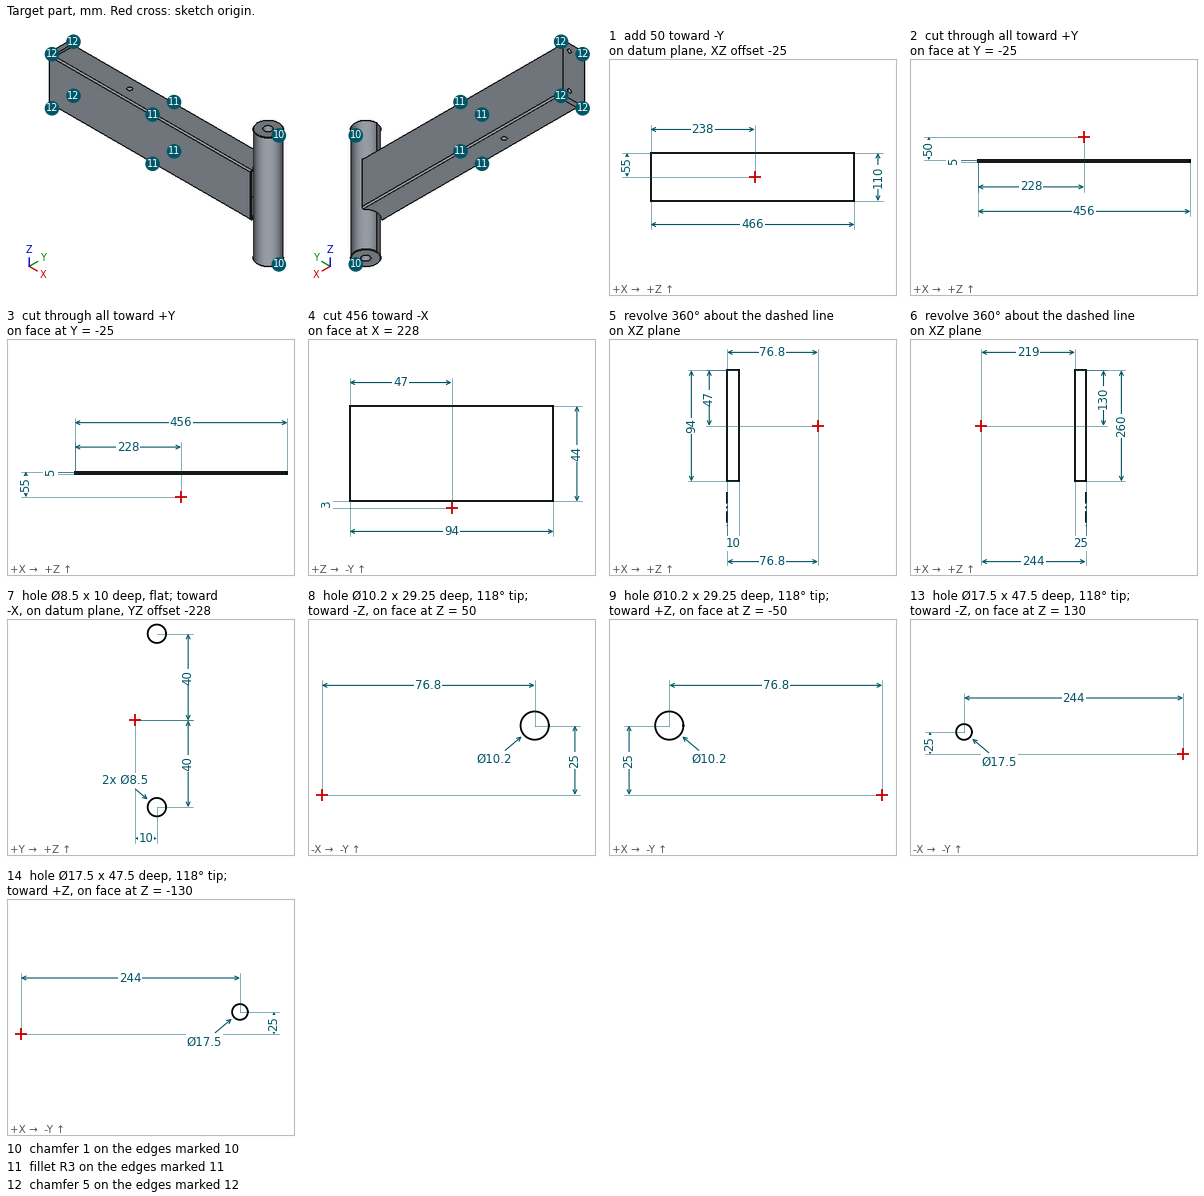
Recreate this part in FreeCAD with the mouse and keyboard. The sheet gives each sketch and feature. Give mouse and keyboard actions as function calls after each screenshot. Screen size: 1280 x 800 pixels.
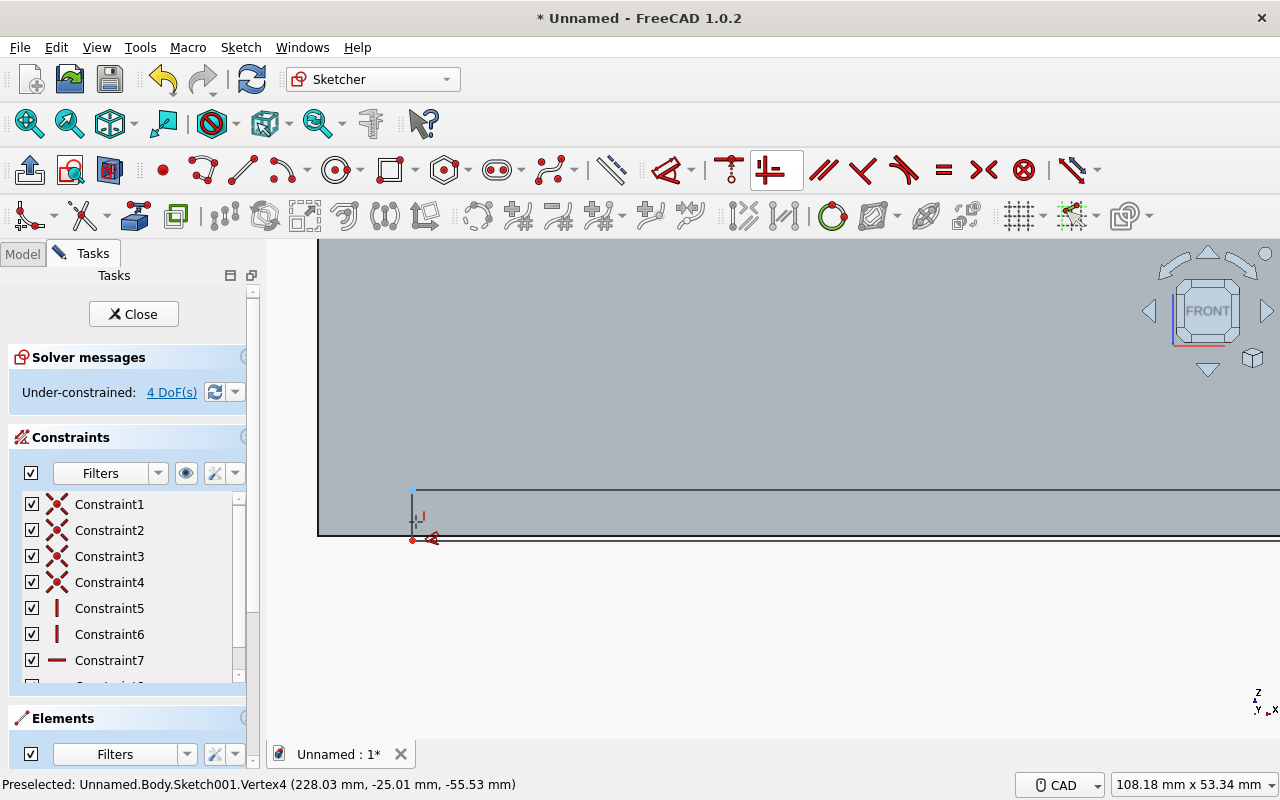
click(412, 515)
click(378, 515)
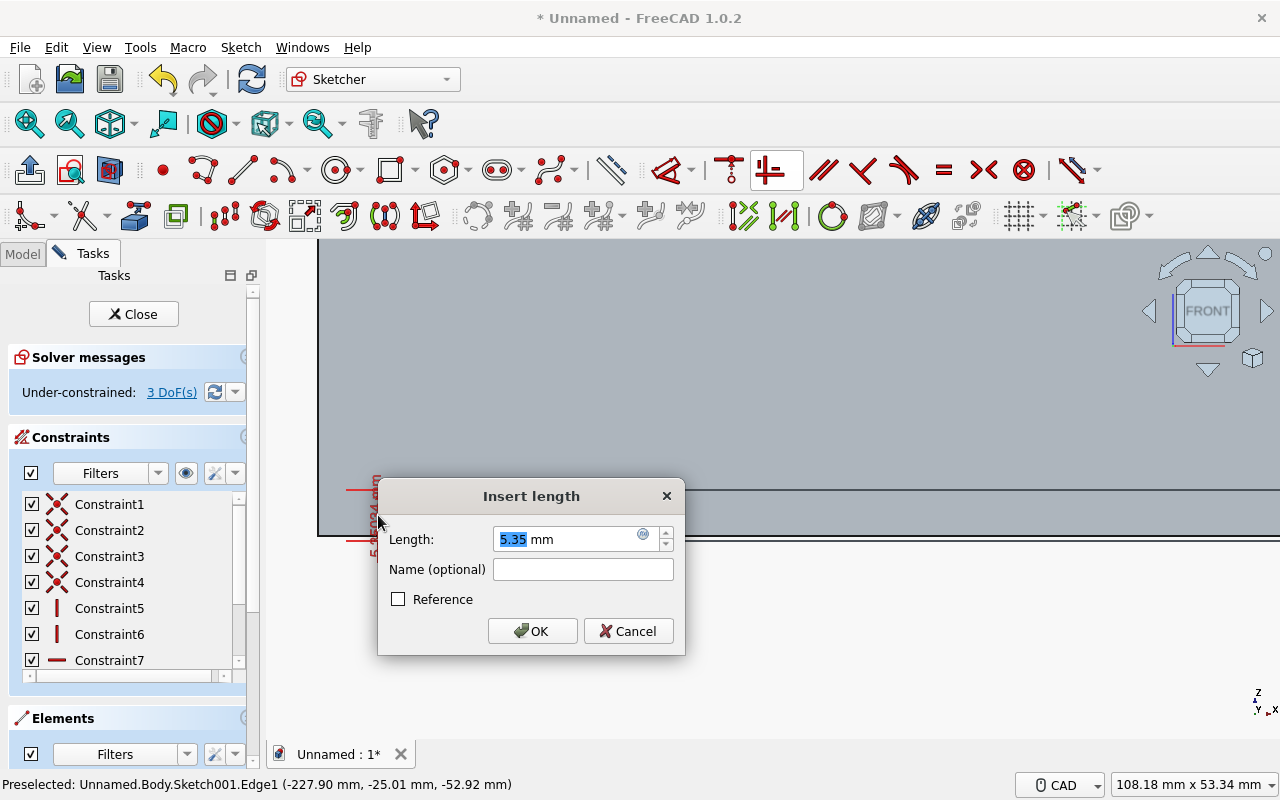
text(5)
key(Return)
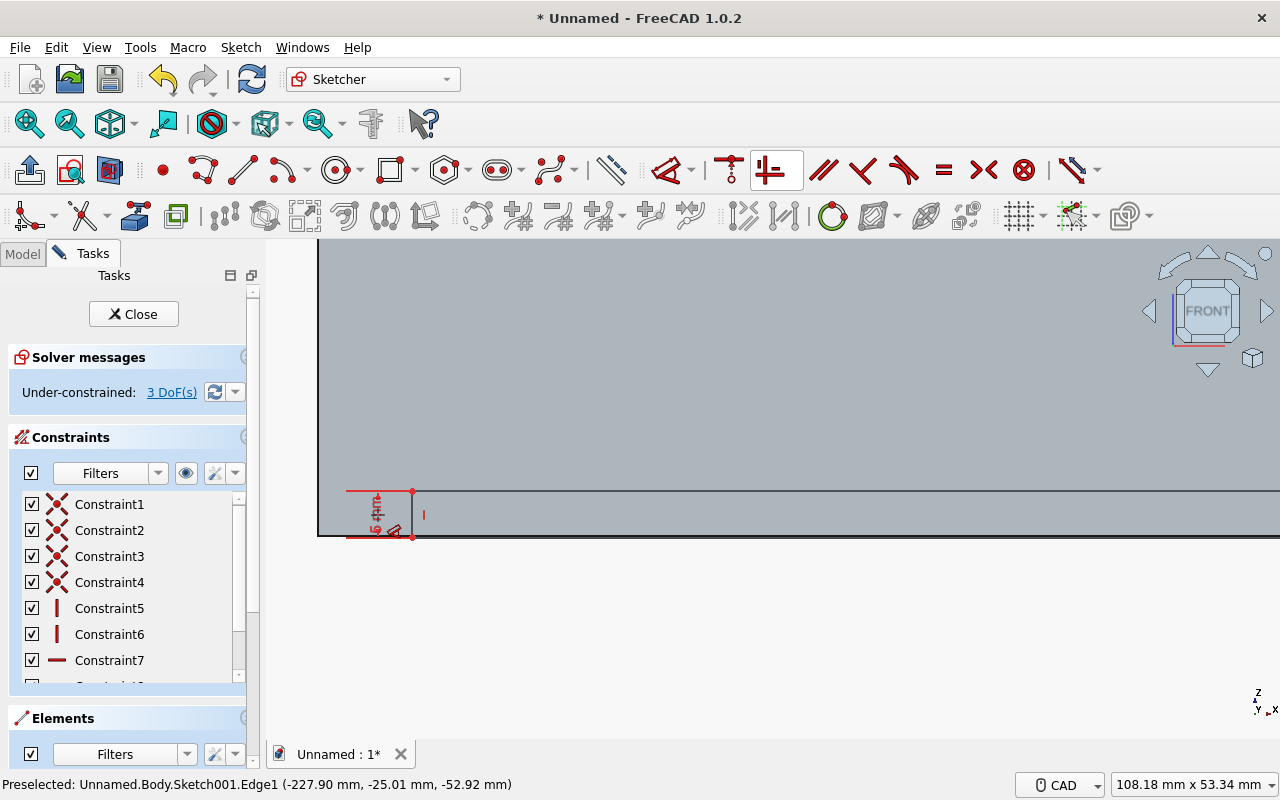
scroll(416, 522, down, 10)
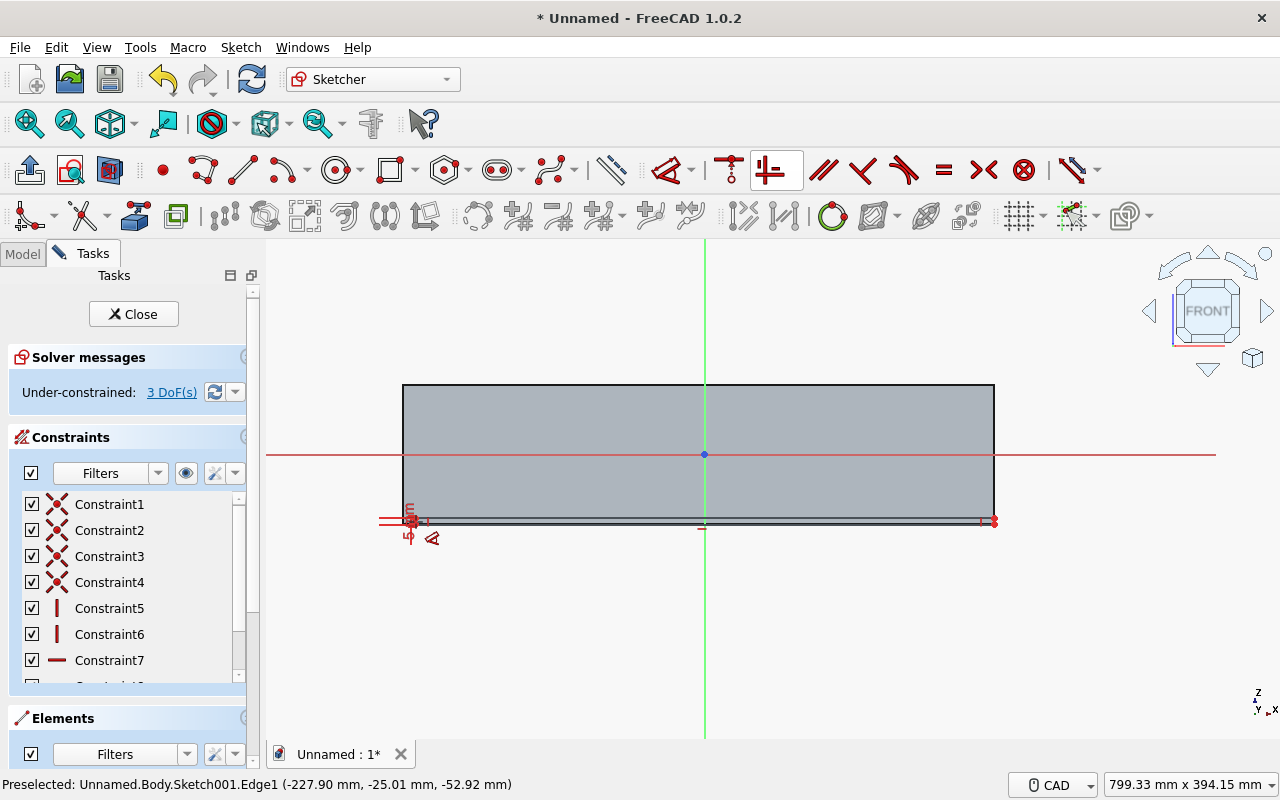
scroll(589, 525, up, 4)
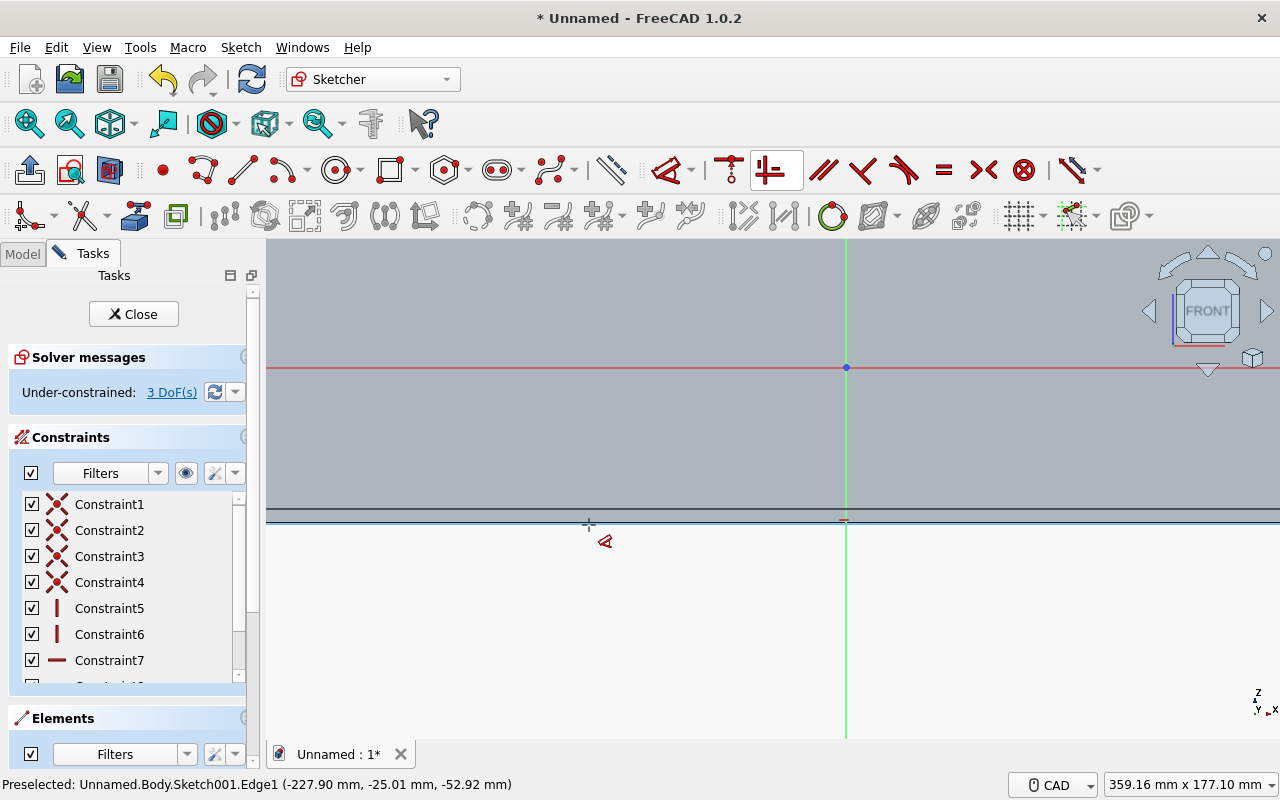
click(589, 524)
click(704, 558)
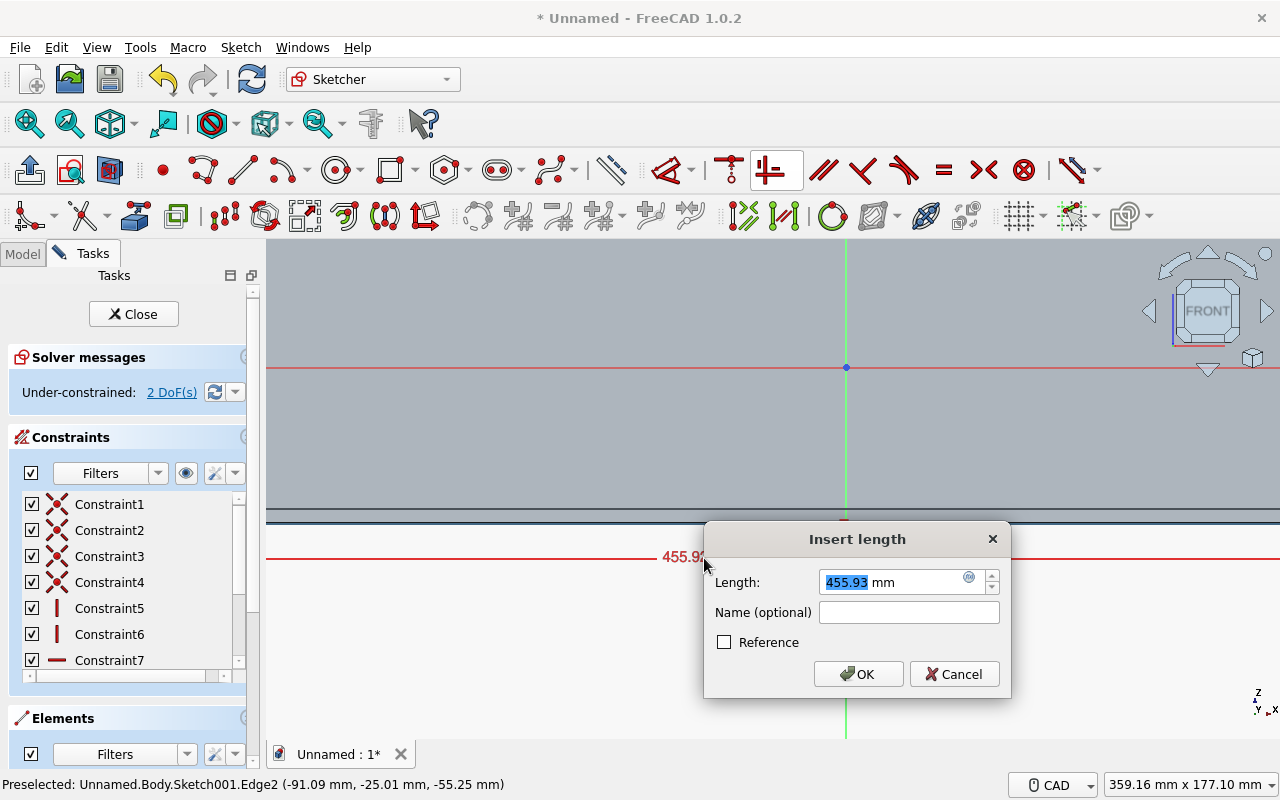
text(456)
key(Return)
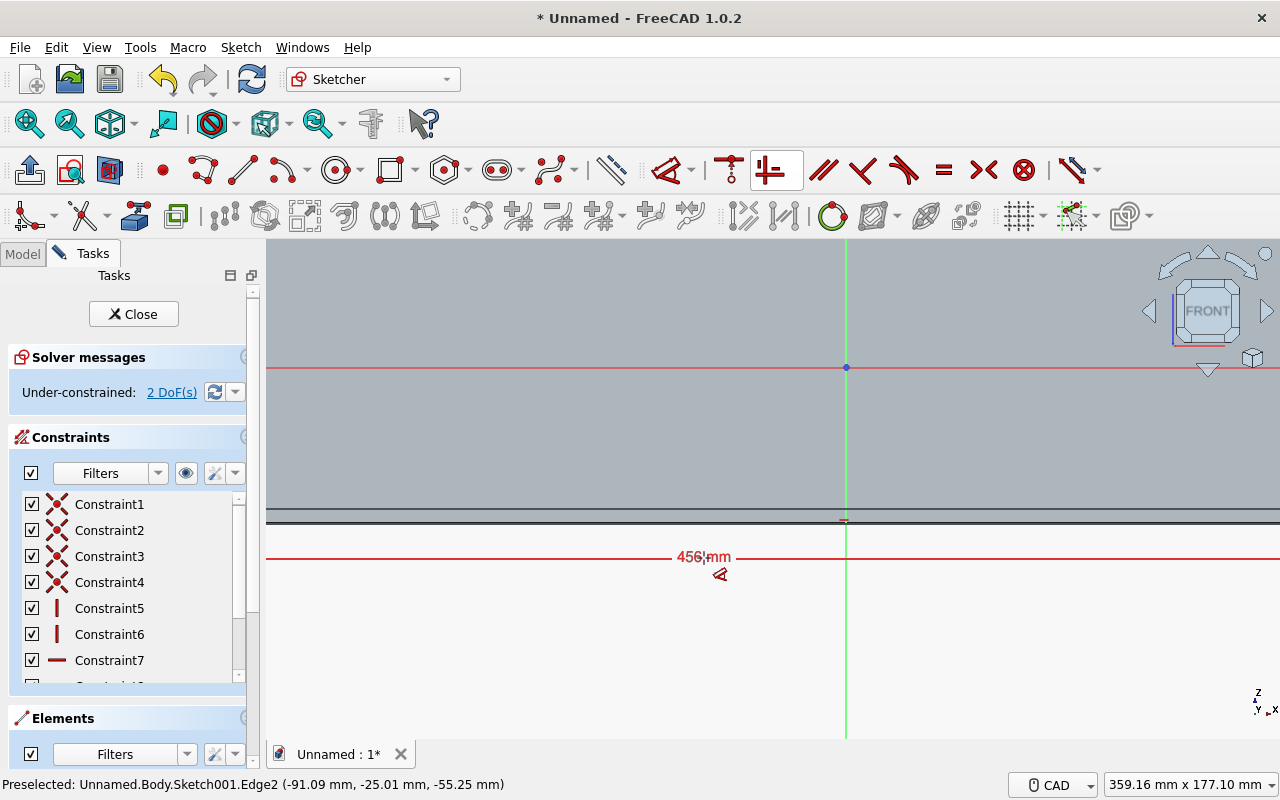
scroll(589, 525, down, 4)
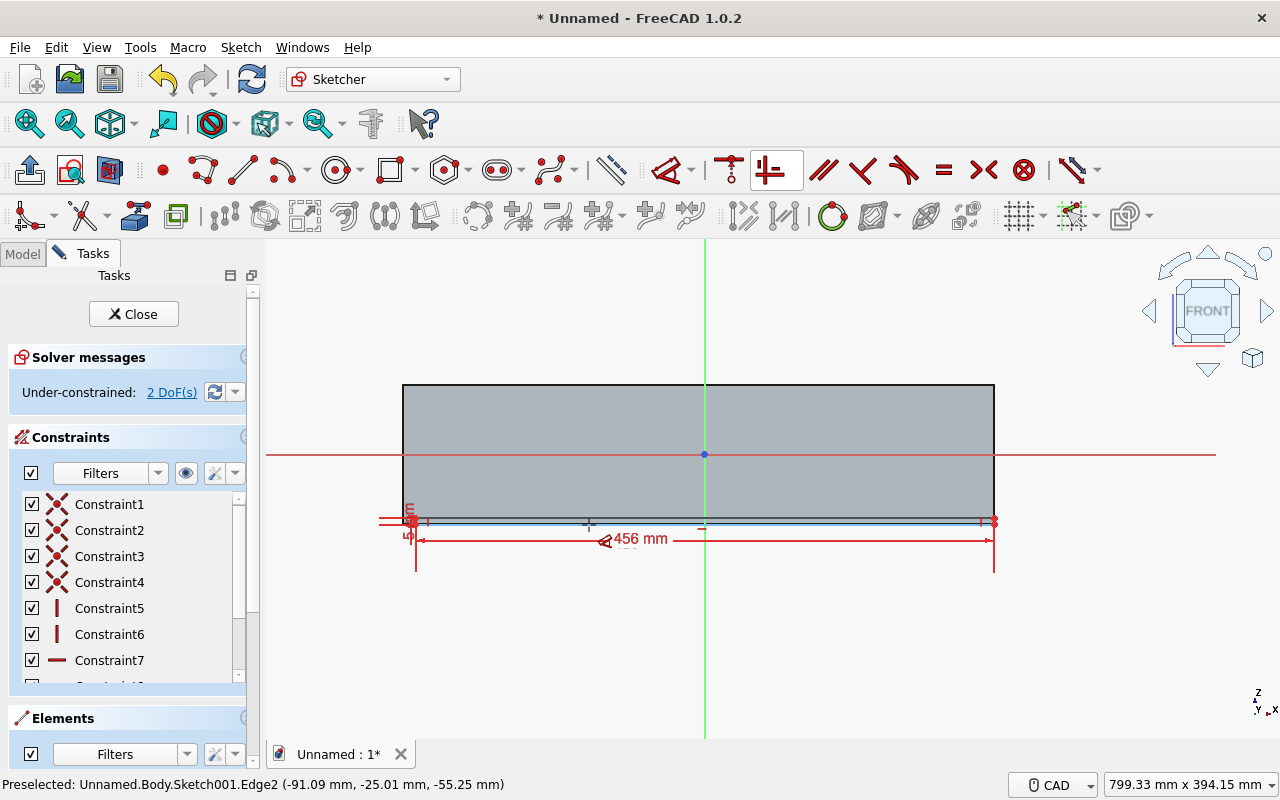
scroll(416, 518, up, 4)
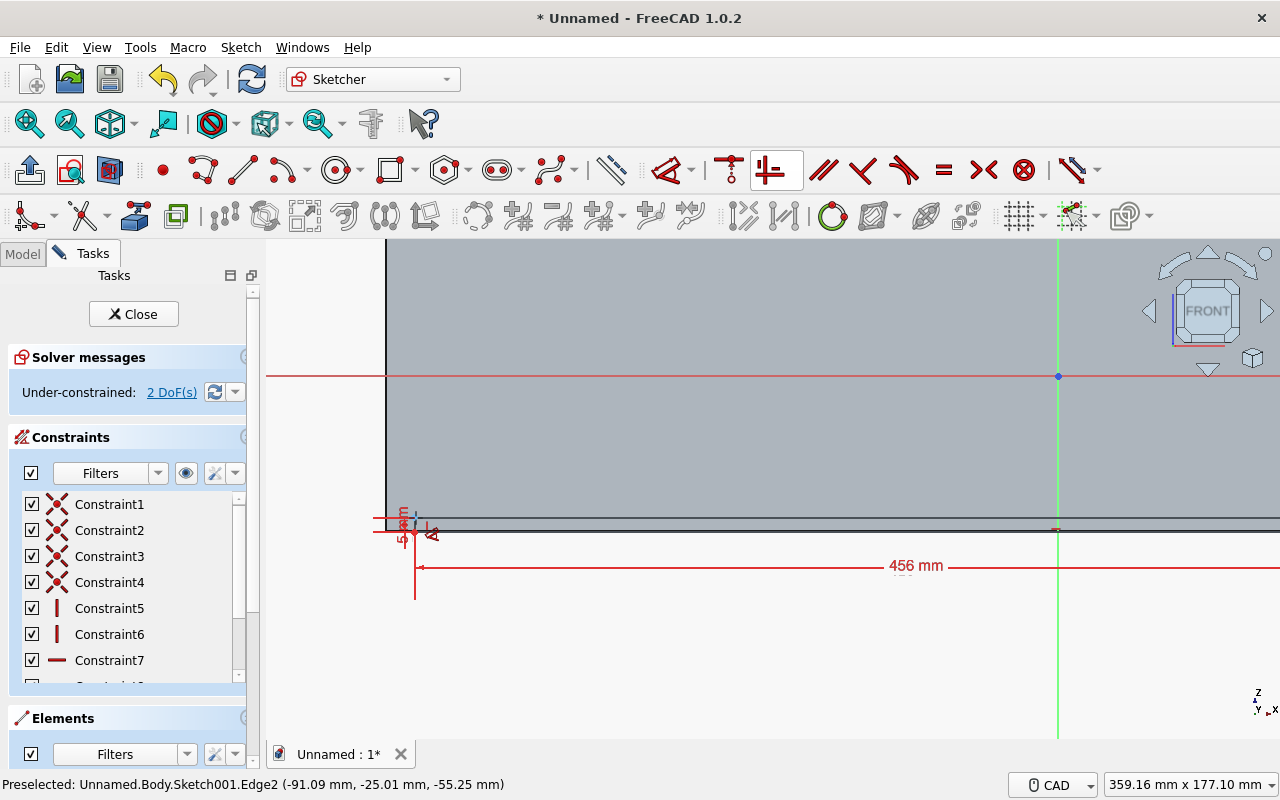
click(415, 518)
click(381, 447)